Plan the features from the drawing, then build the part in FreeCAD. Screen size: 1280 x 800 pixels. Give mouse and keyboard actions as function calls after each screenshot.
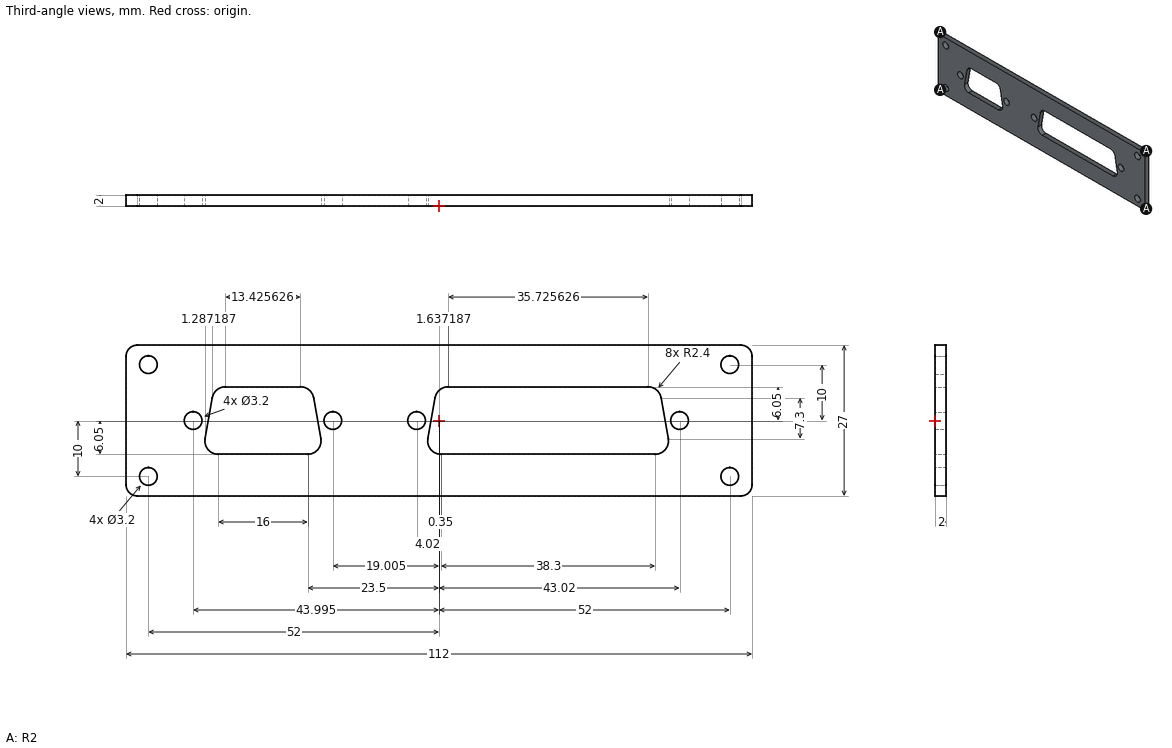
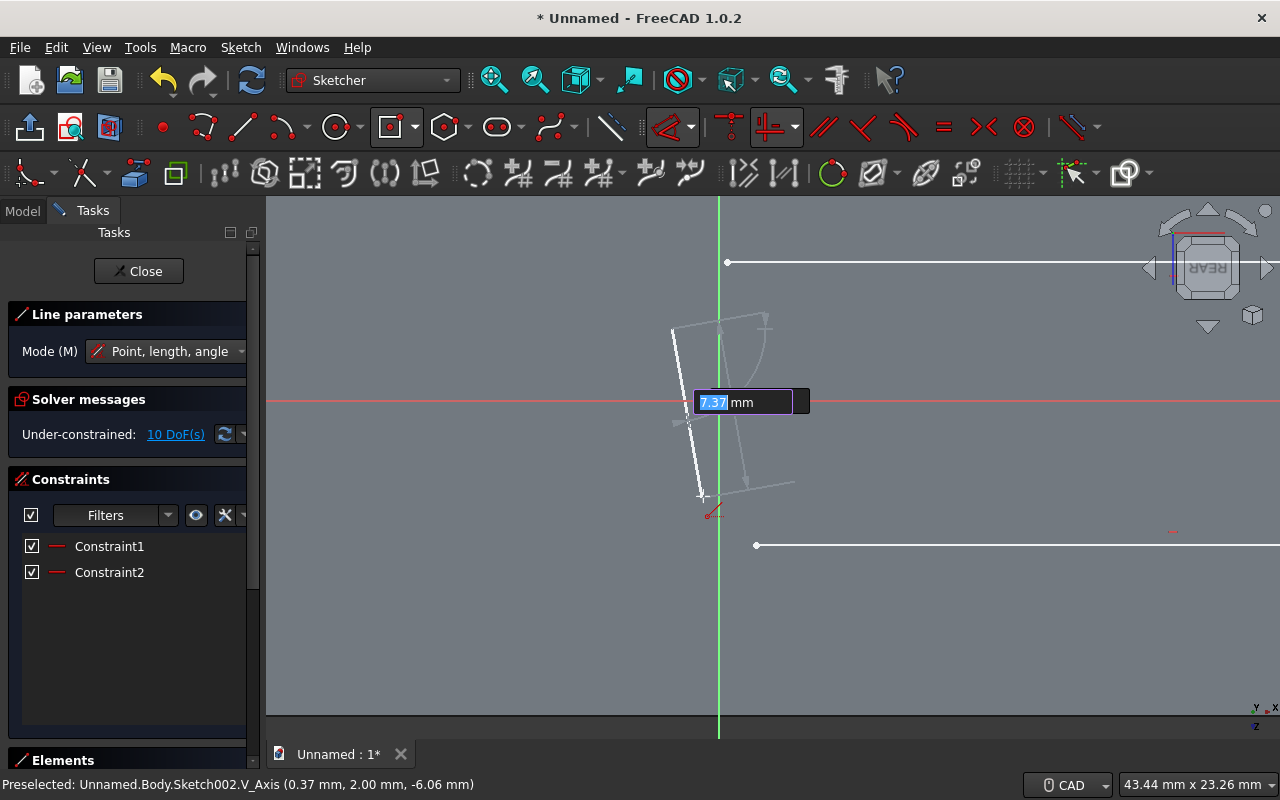
click(702, 496)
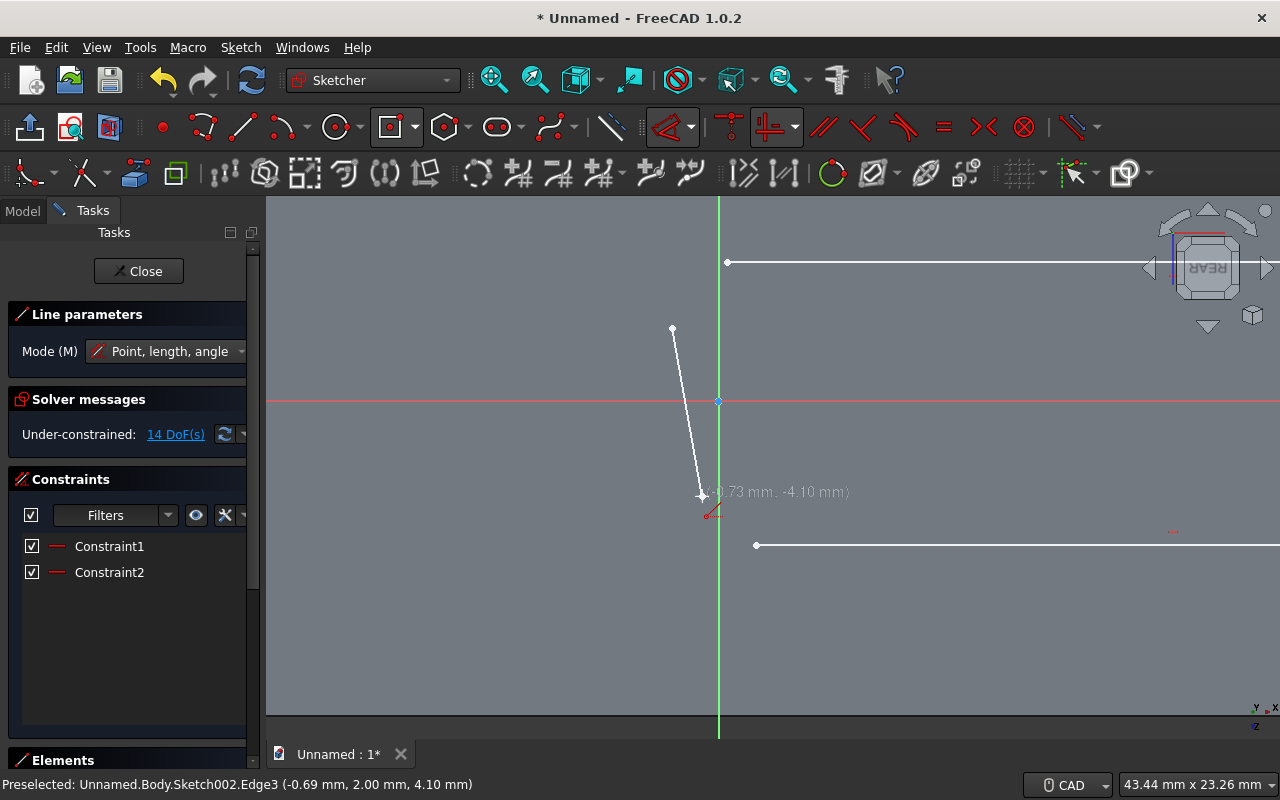
key(g)
key(3)
key(a)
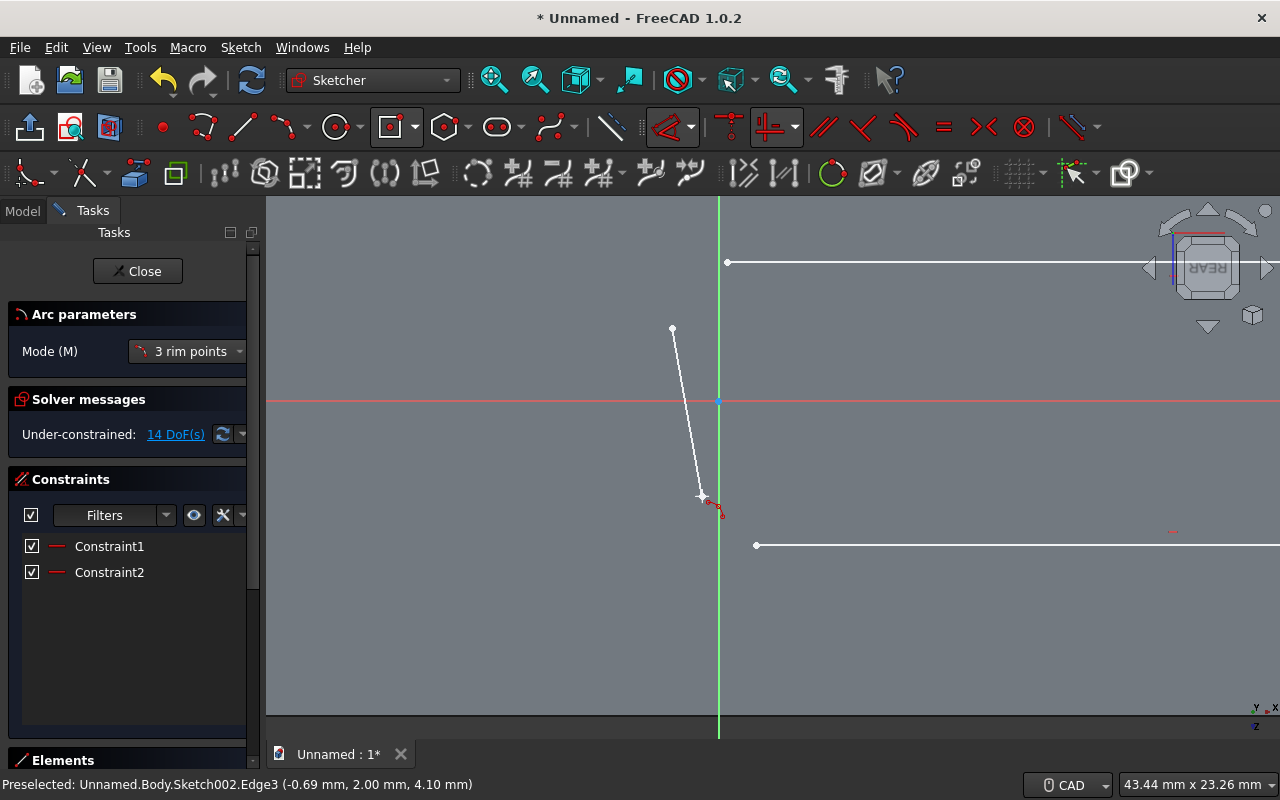
scroll(703, 496, down, 6)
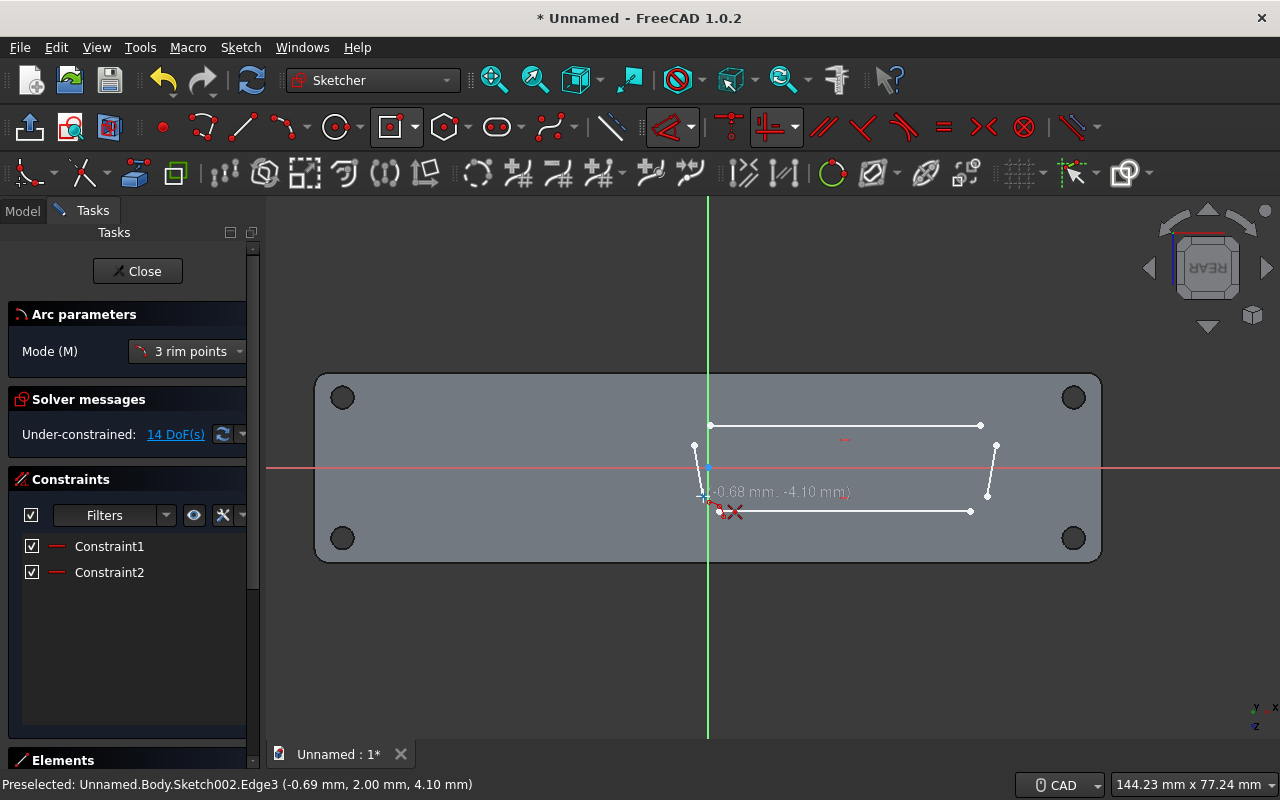
click(971, 511)
click(987, 497)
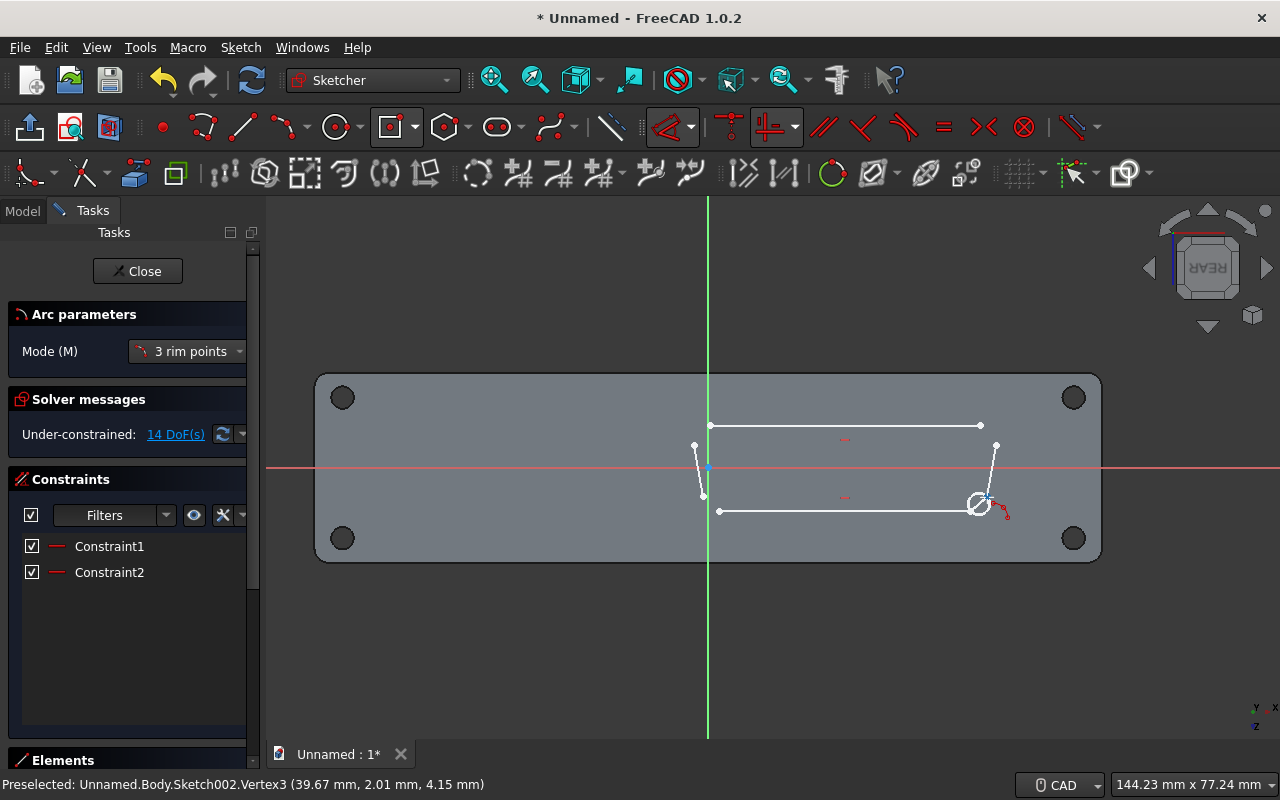
scroll(982, 506, up, 7)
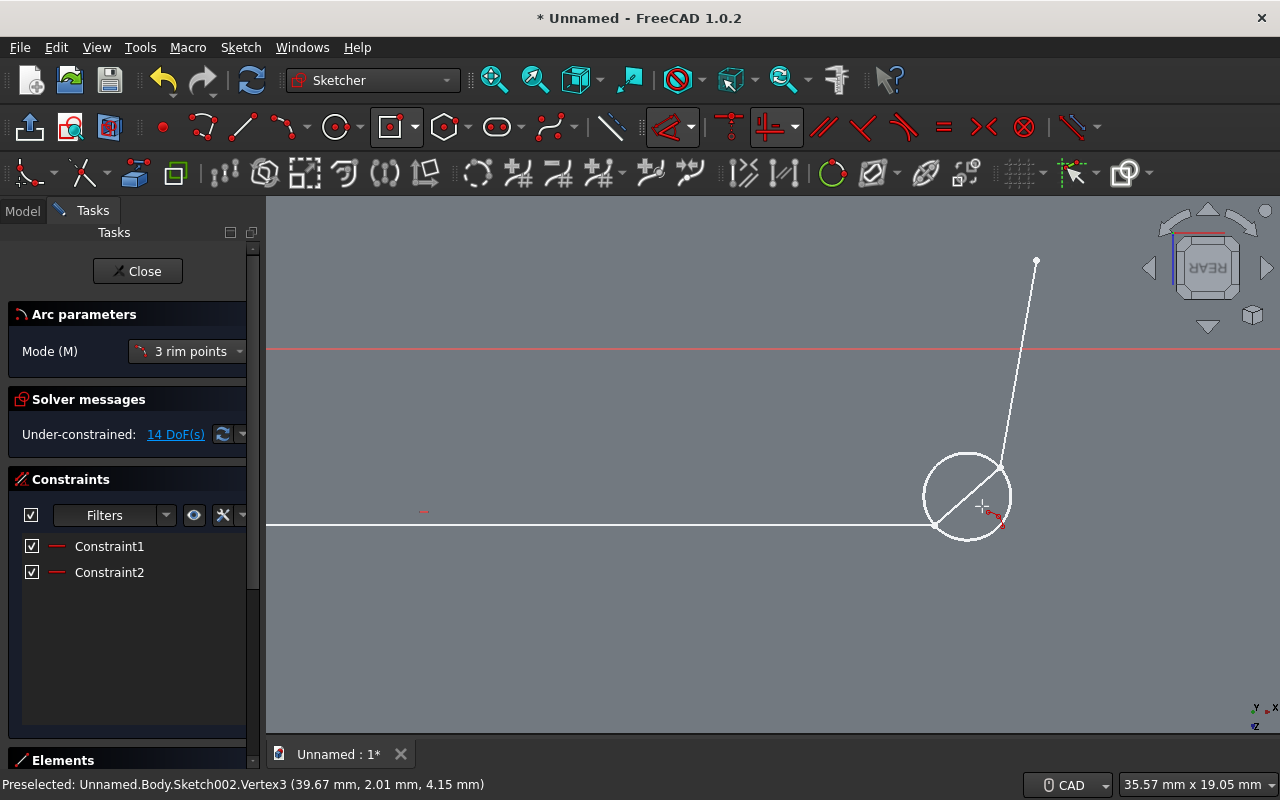
click(978, 506)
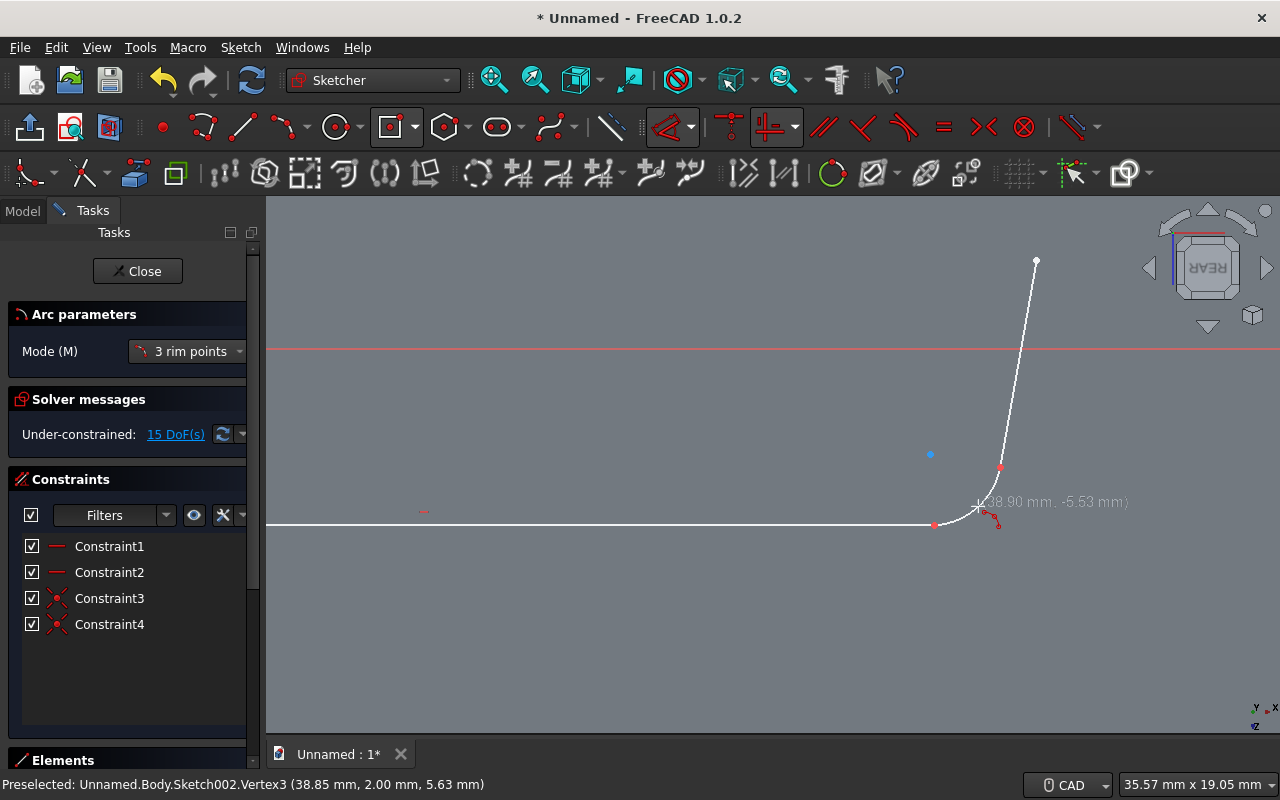
scroll(982, 506, down, 7)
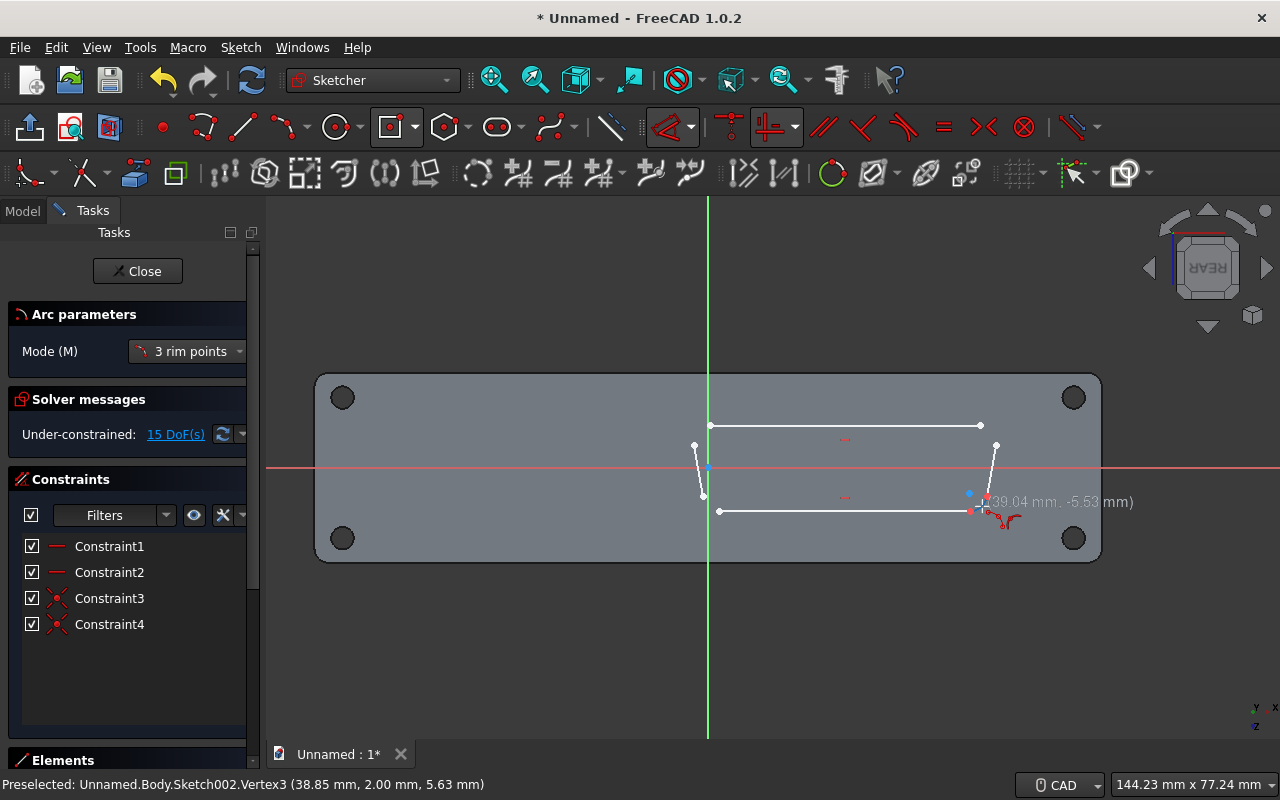
click(996, 446)
click(980, 426)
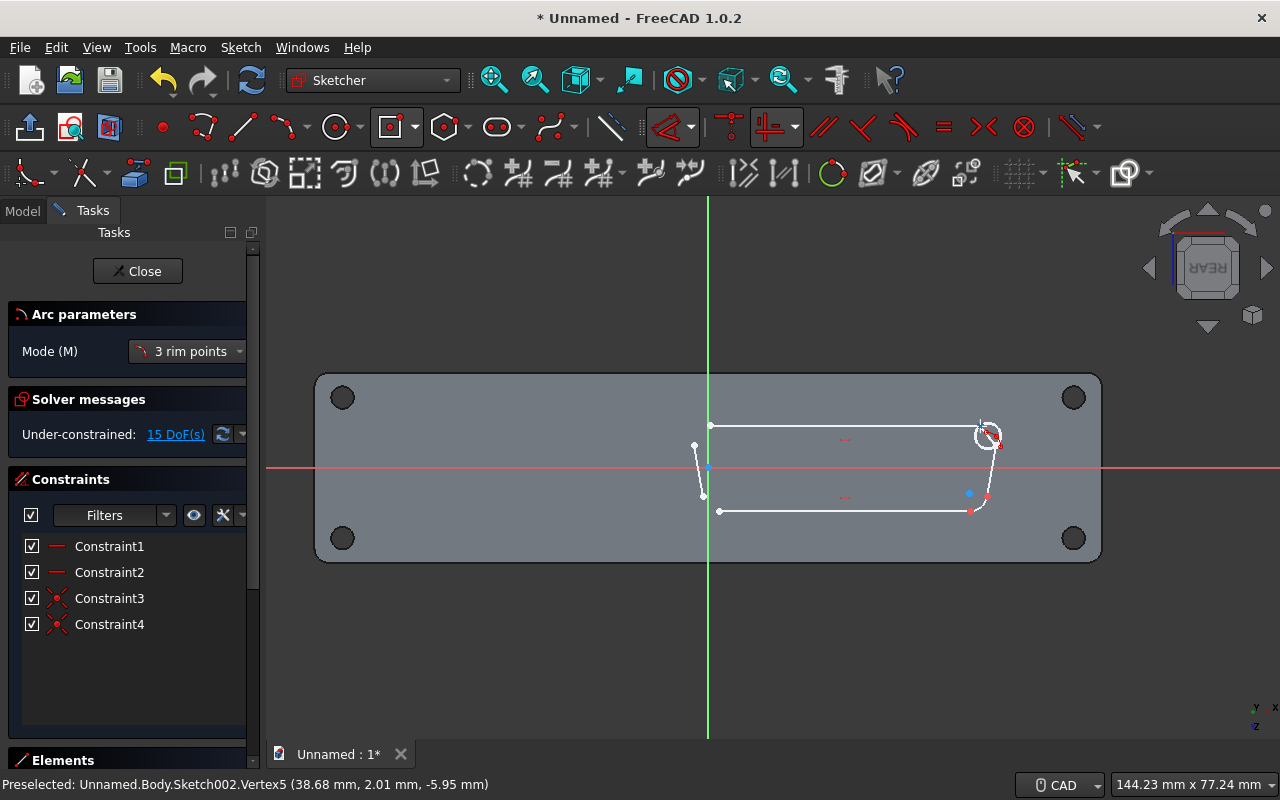
scroll(993, 431, up, 5)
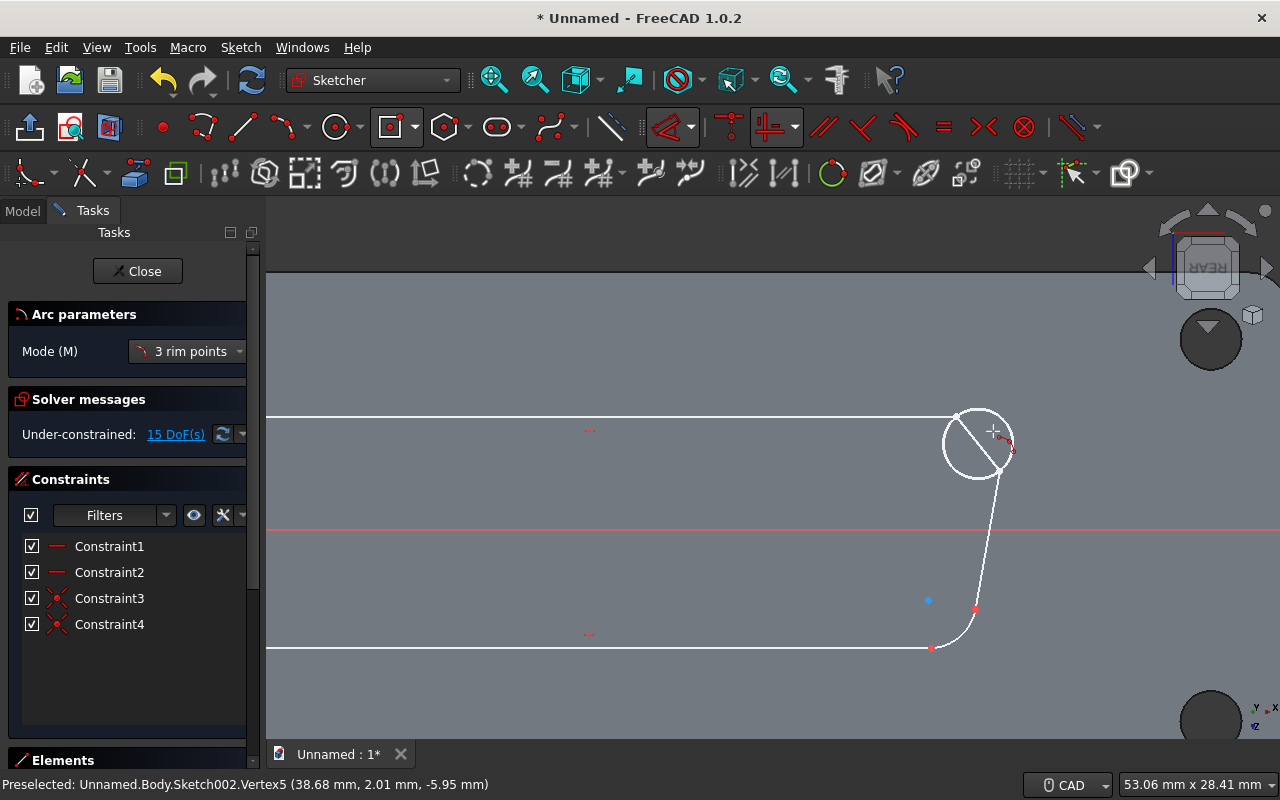
click(991, 431)